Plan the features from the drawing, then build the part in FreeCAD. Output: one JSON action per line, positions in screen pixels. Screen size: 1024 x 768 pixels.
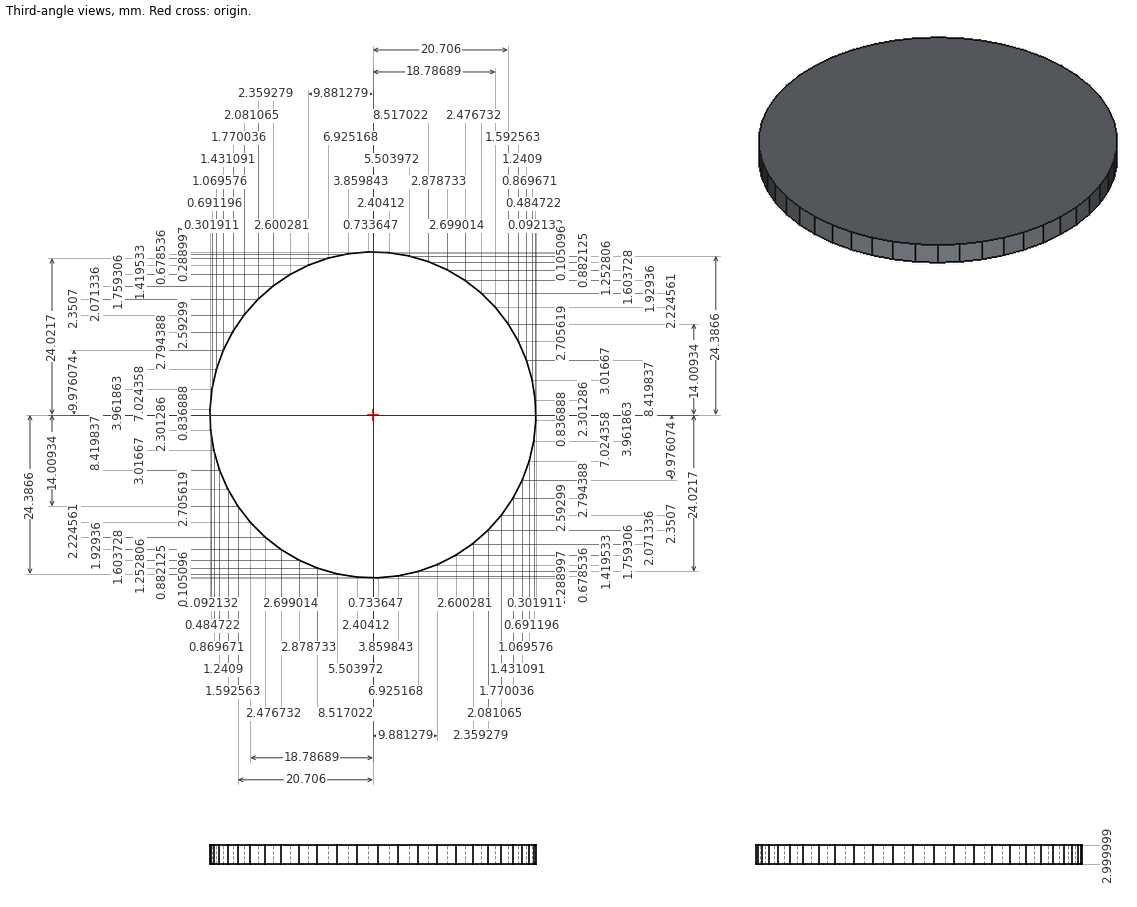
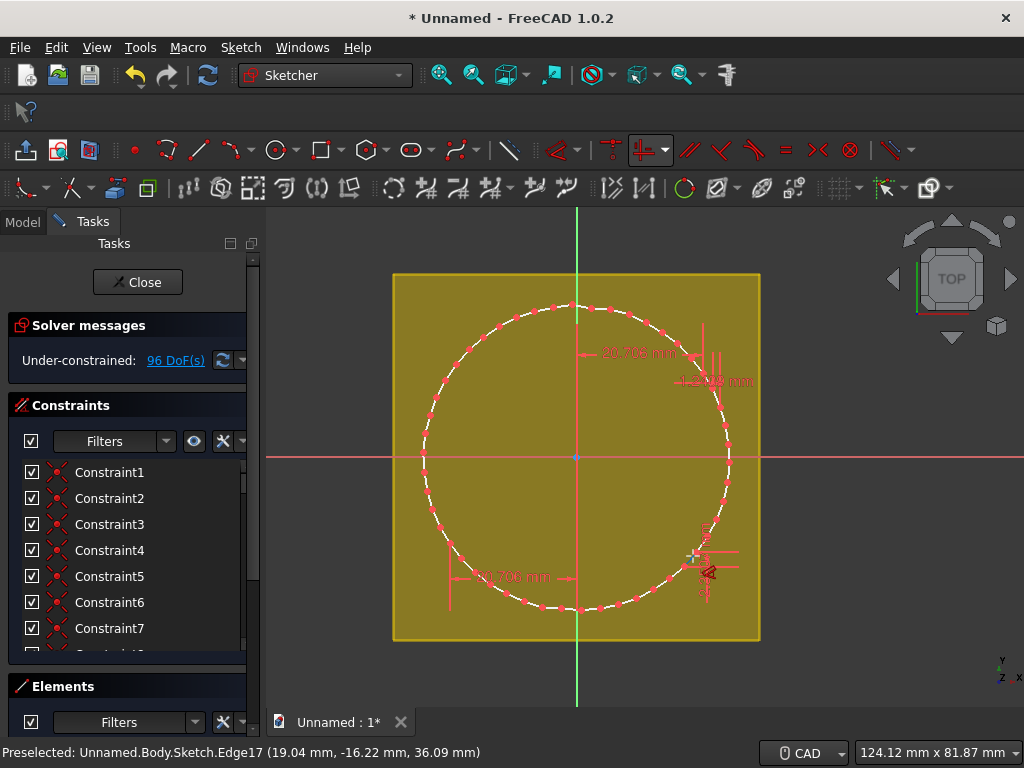
{"action": "scroll", "coordinate": [438, 522], "scroll_direction": "up", "scroll_amount": 9}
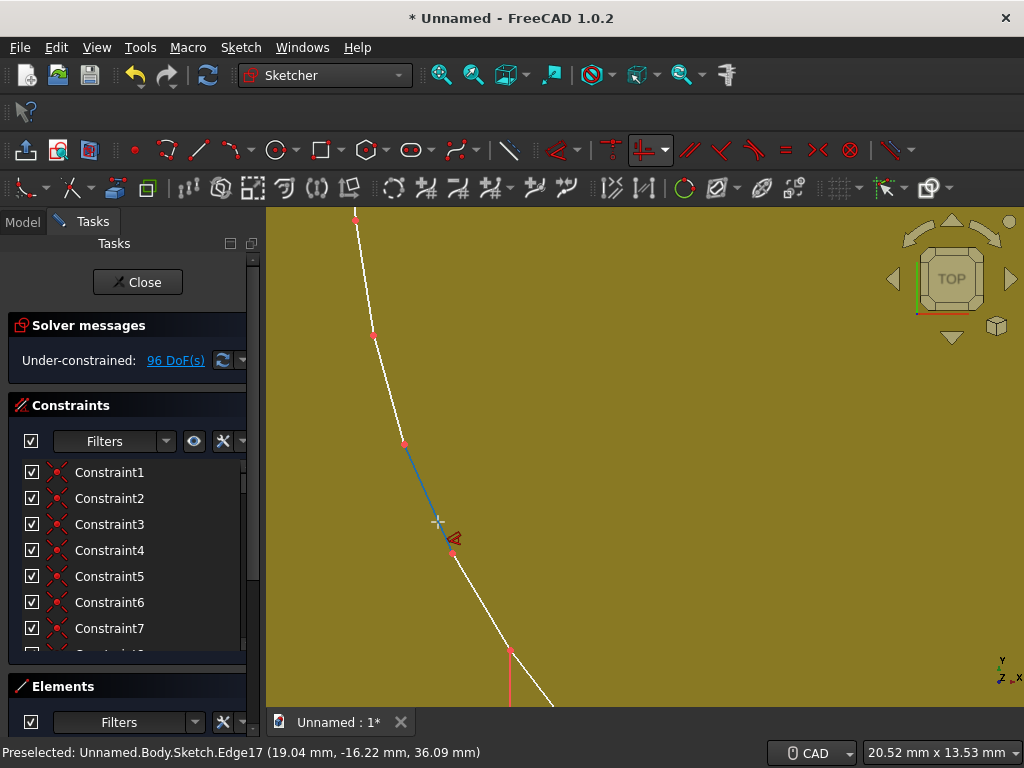
{"action": "left_click", "coordinate": [438, 521]}
{"action": "left_click", "coordinate": [428, 587]}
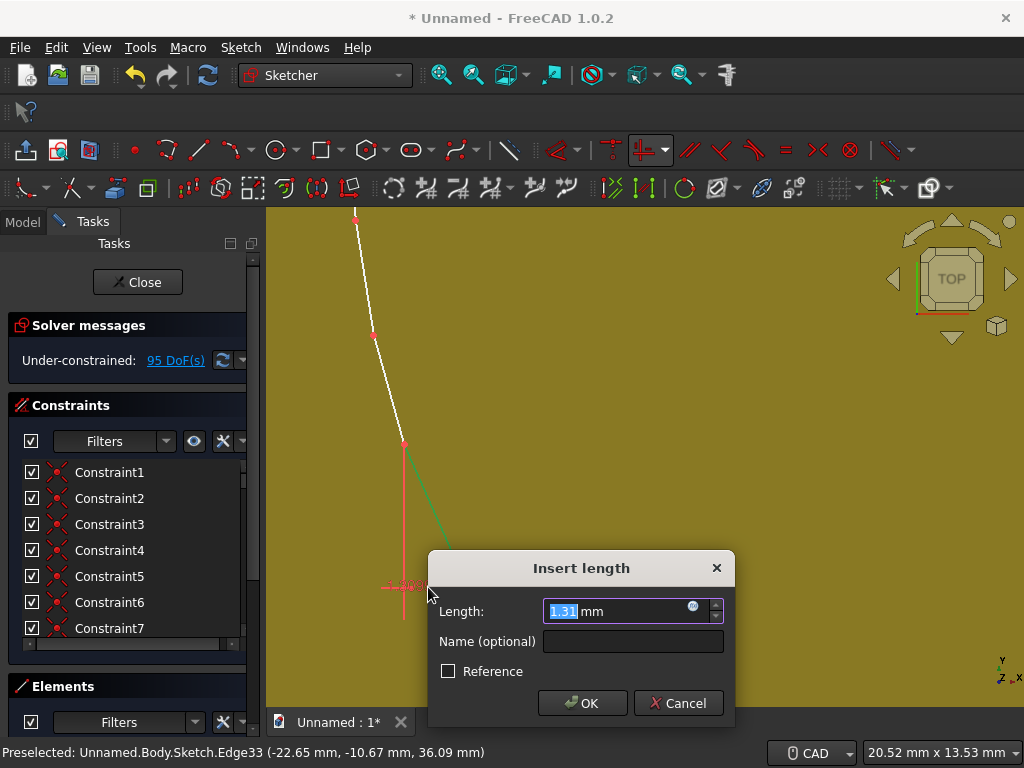
{"action": "type", "text": "1.2409"}
{"action": "key", "text": "Return"}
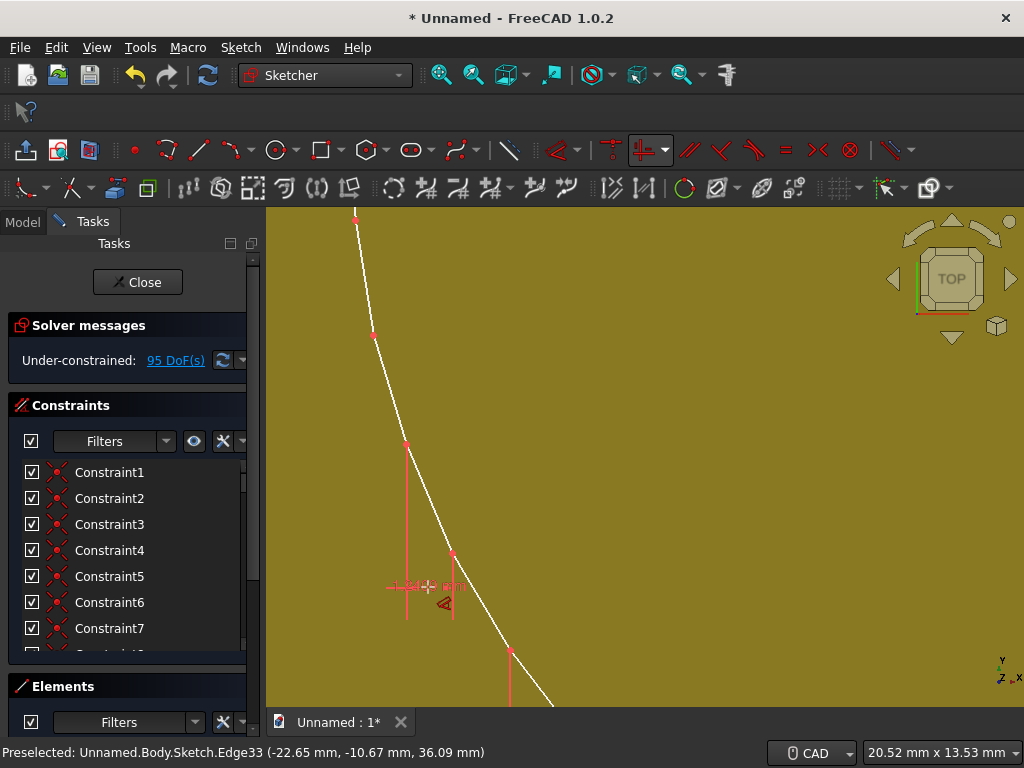
{"action": "scroll", "coordinate": [438, 522], "scroll_direction": "down", "scroll_amount": 9}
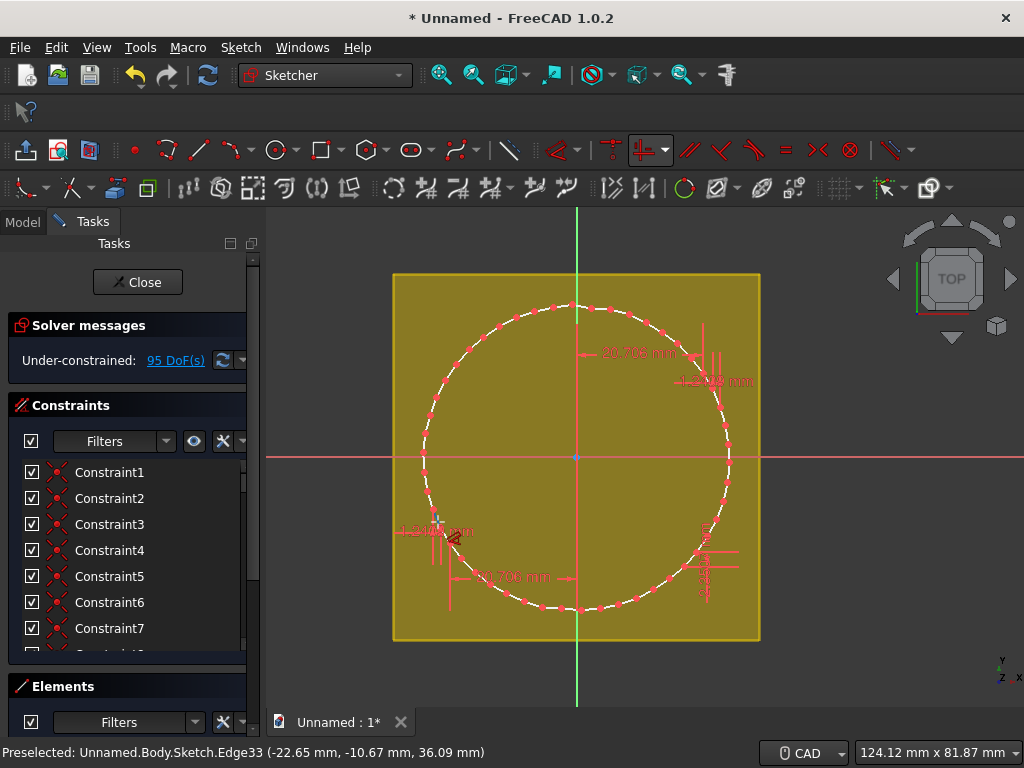
{"action": "scroll", "coordinate": [460, 360], "scroll_direction": "up", "scroll_amount": 6}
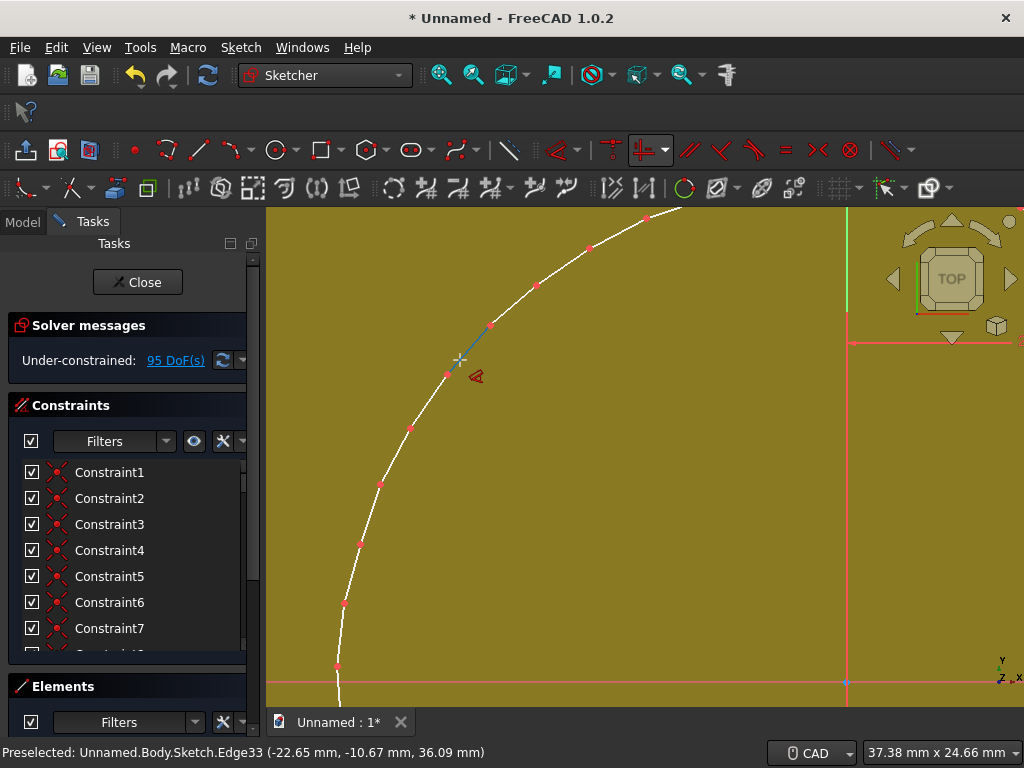
{"action": "left_click", "coordinate": [460, 360]}
{"action": "left_click", "coordinate": [413, 350]}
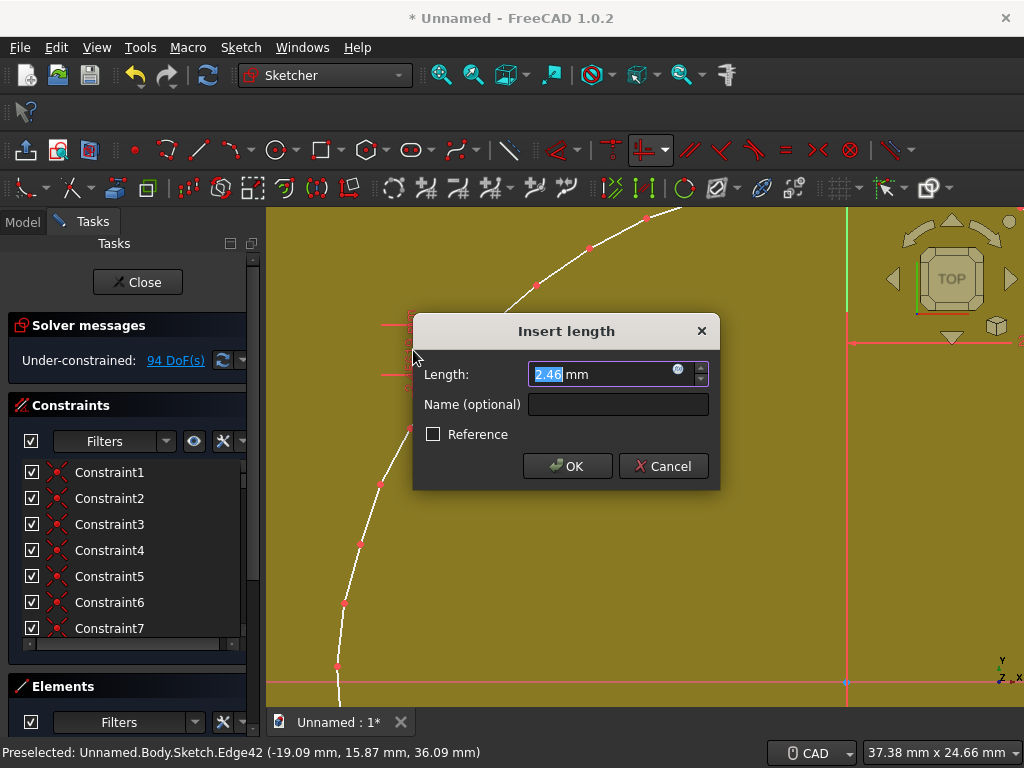
{"action": "type", "text": "2.3507"}
{"action": "key", "text": "Return"}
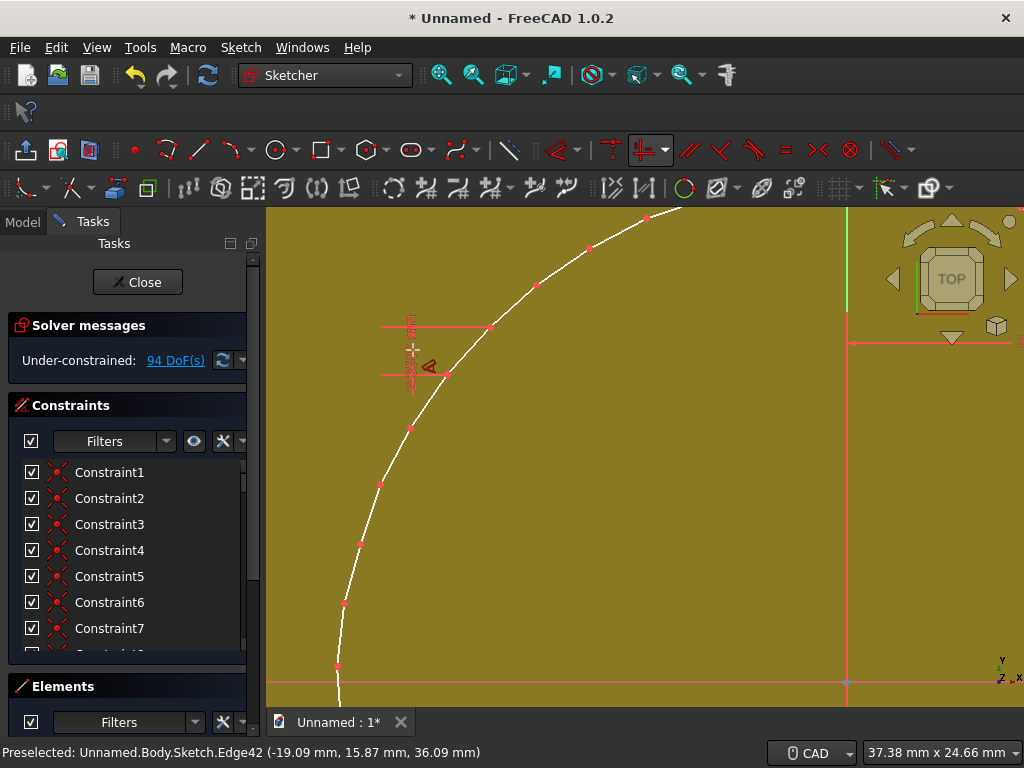
{"action": "scroll", "coordinate": [460, 360], "scroll_direction": "down", "scroll_amount": 6}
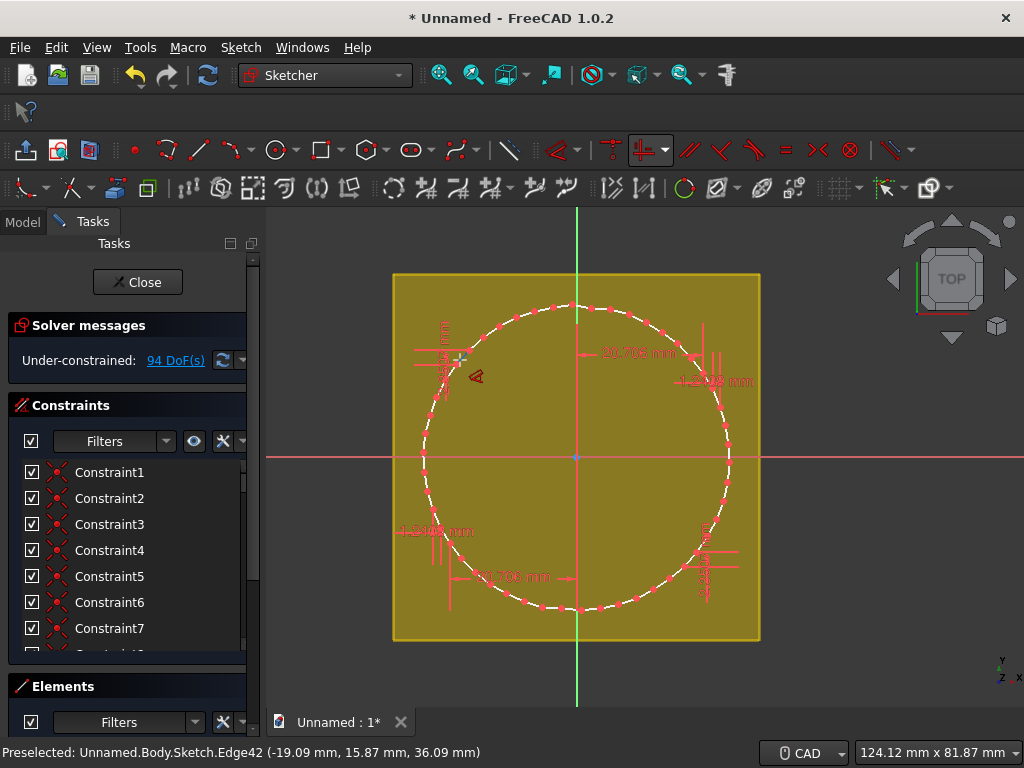
{"action": "left_click", "coordinate": [611, 310]}
{"action": "left_click", "coordinate": [645, 383]}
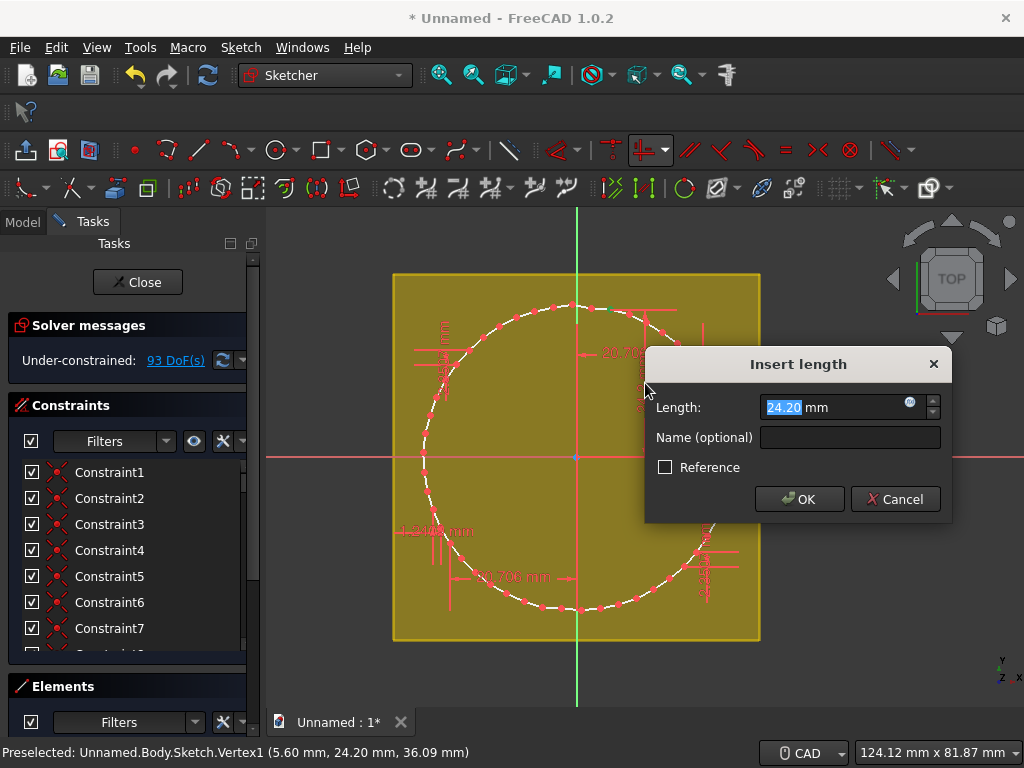
{"action": "type", "text": "24.3866"}
{"action": "key", "text": "Return"}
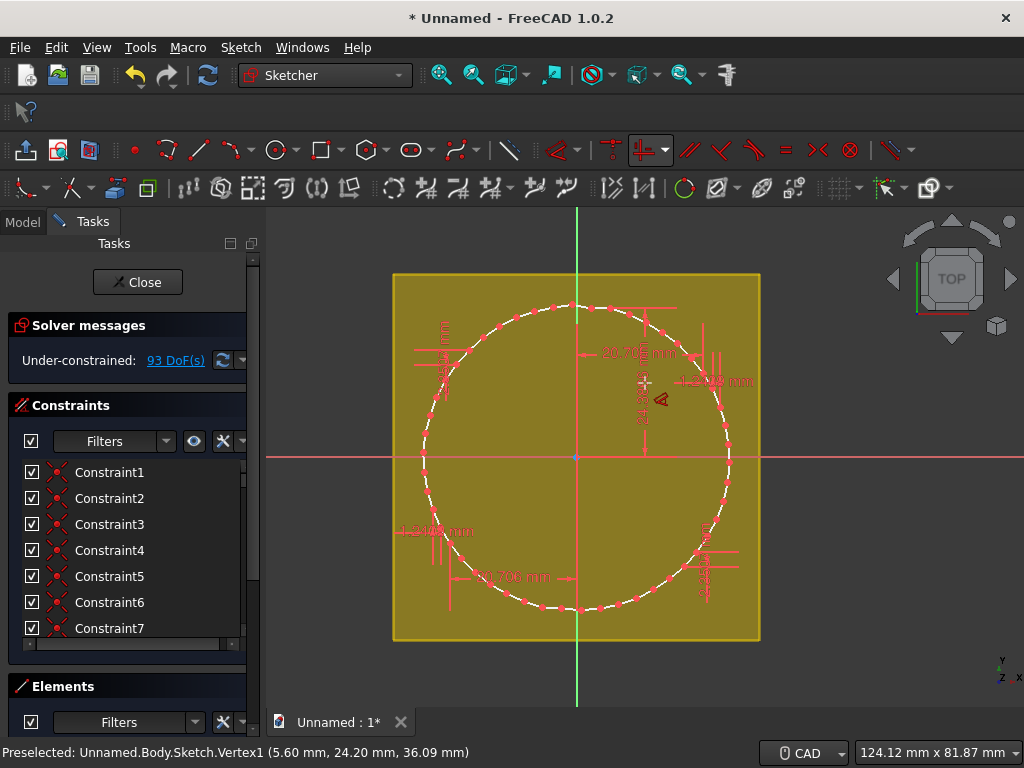
{"action": "left_click", "coordinate": [619, 605]}
{"action": "left_click", "coordinate": [653, 531]}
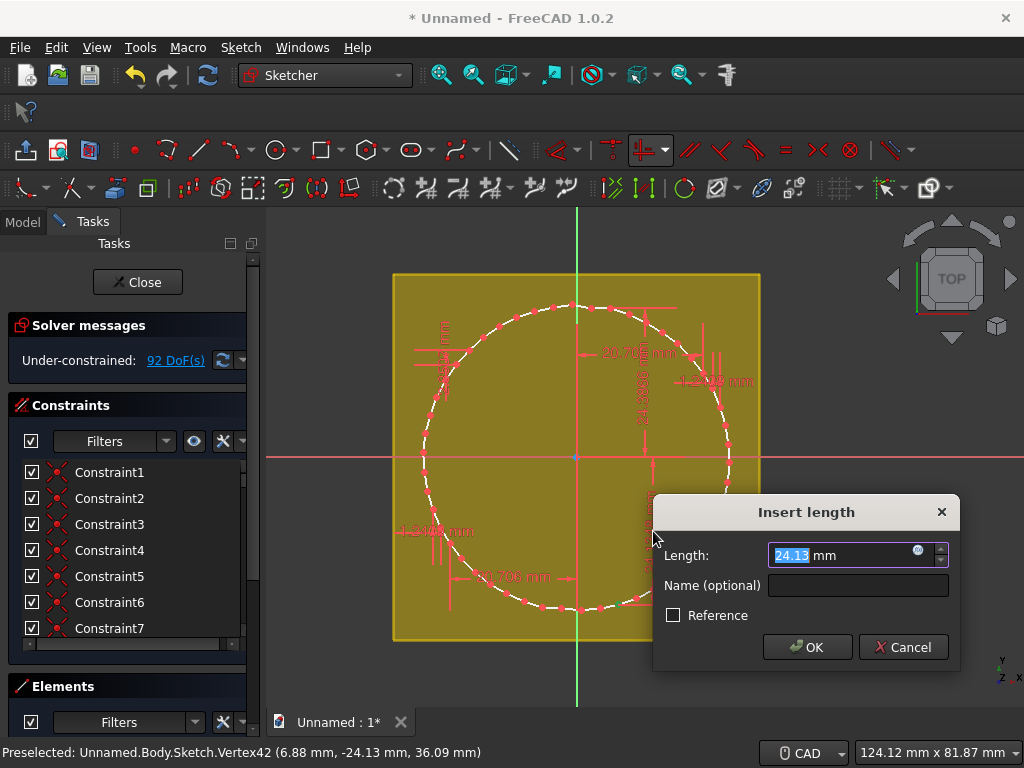
{"action": "type", "text": "24.0217"}
{"action": "key", "text": "Return"}